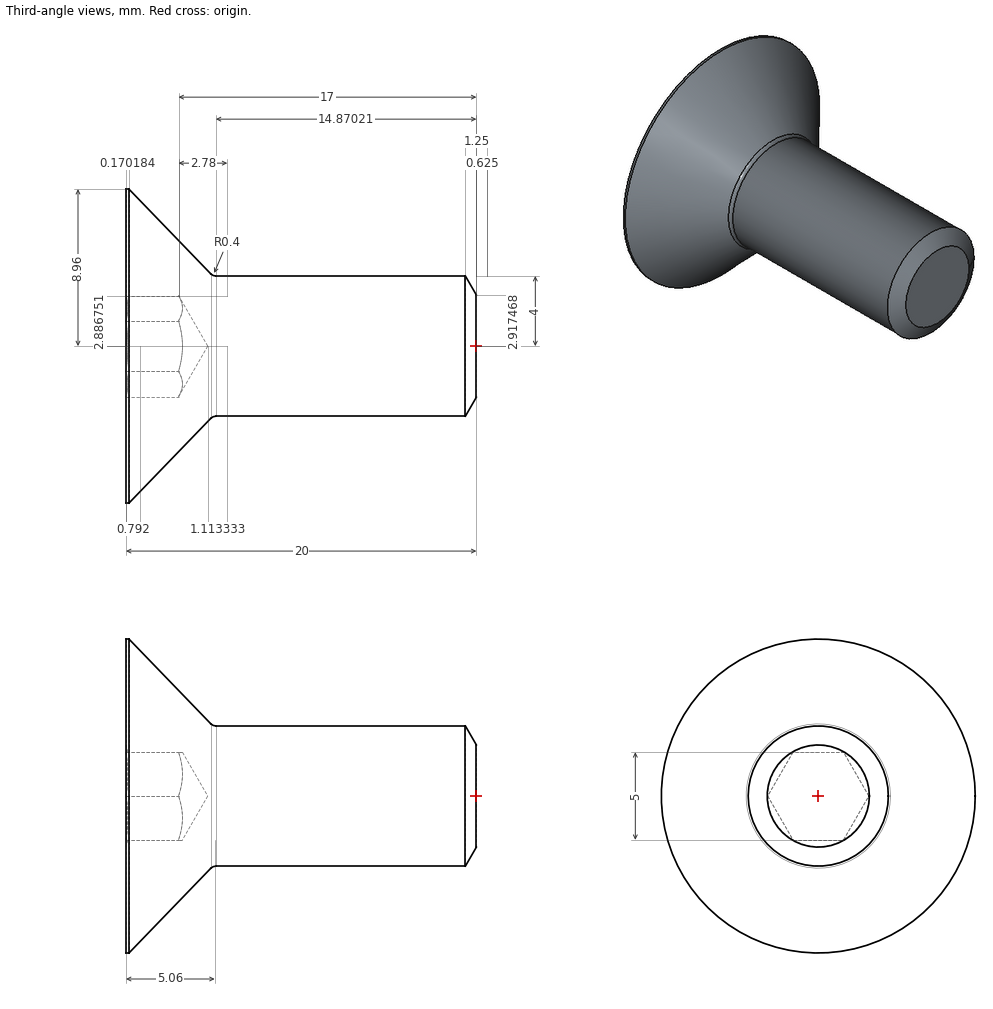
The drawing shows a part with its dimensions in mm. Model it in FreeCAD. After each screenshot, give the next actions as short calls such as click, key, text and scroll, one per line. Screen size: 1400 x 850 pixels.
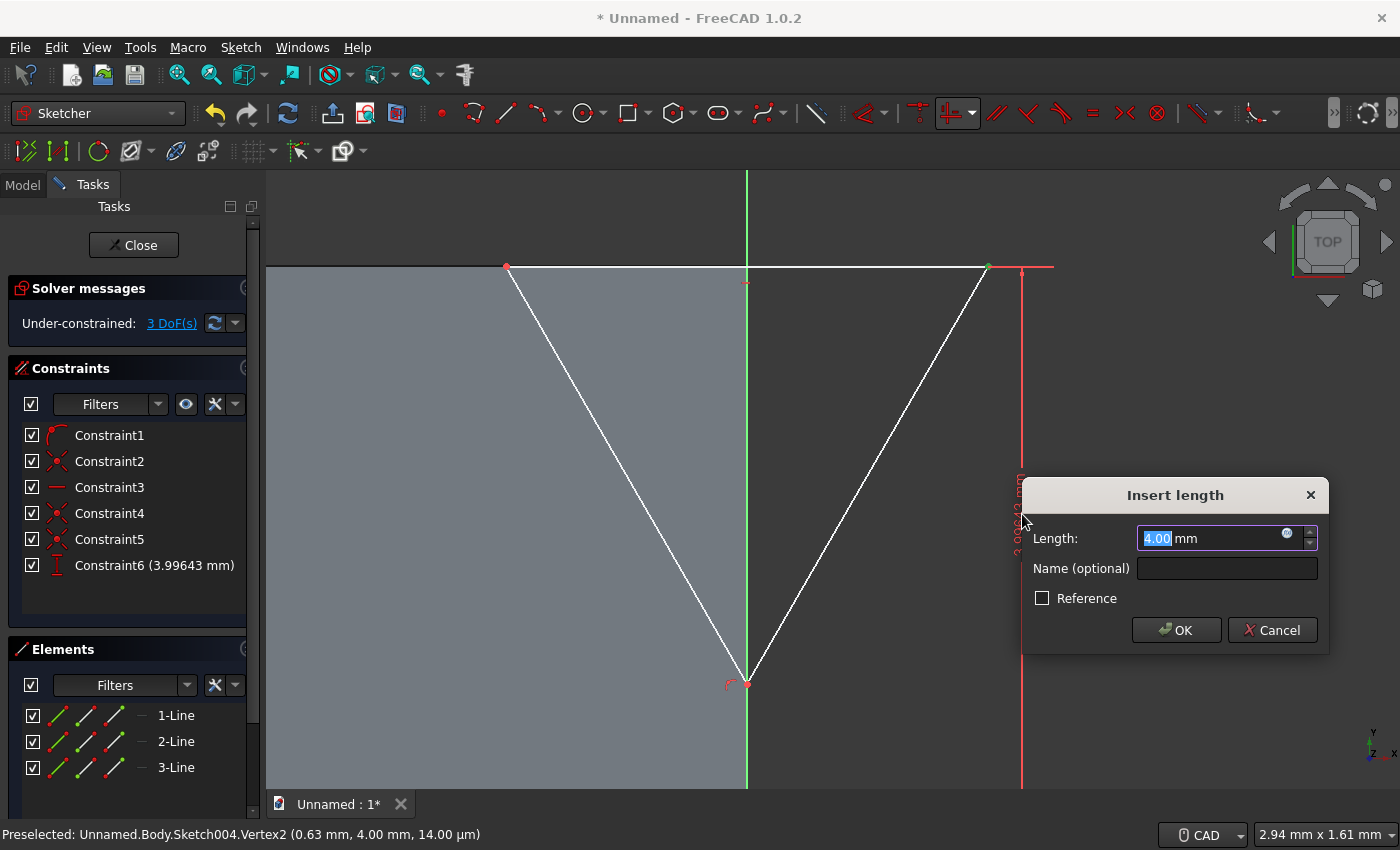
text(4)
key(Return)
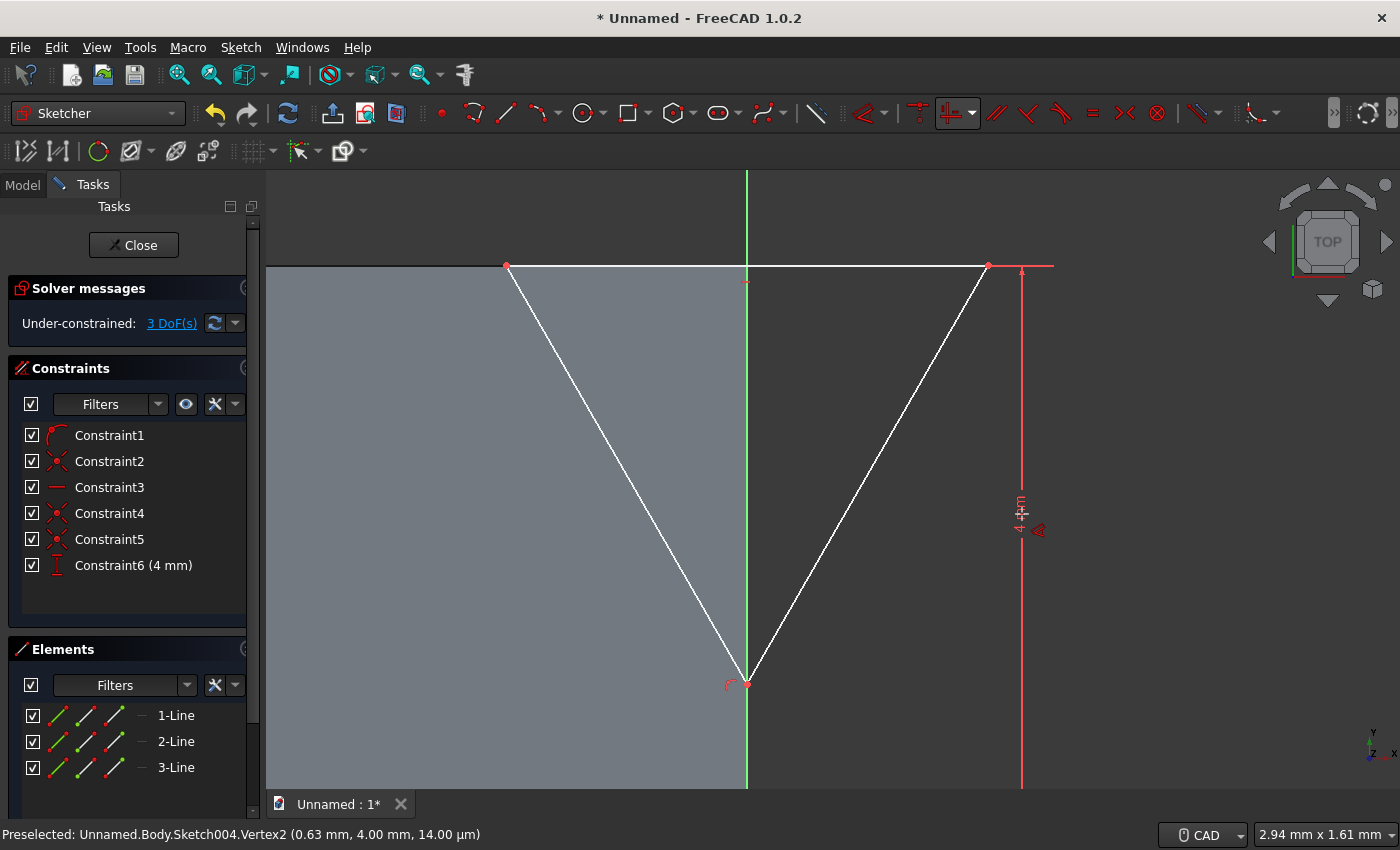
click(843, 266)
click(636, 232)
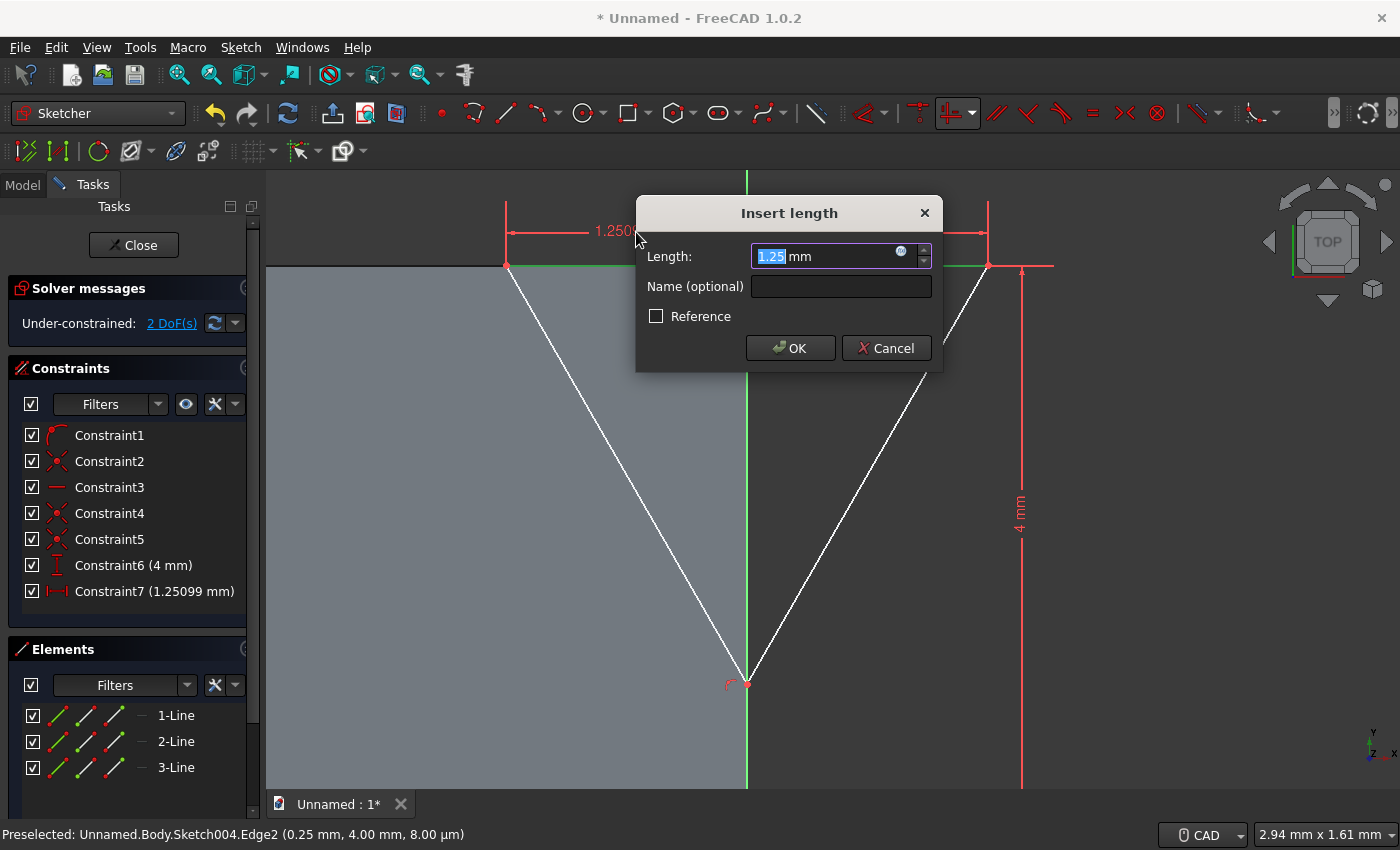
text(1.25)
key(Return)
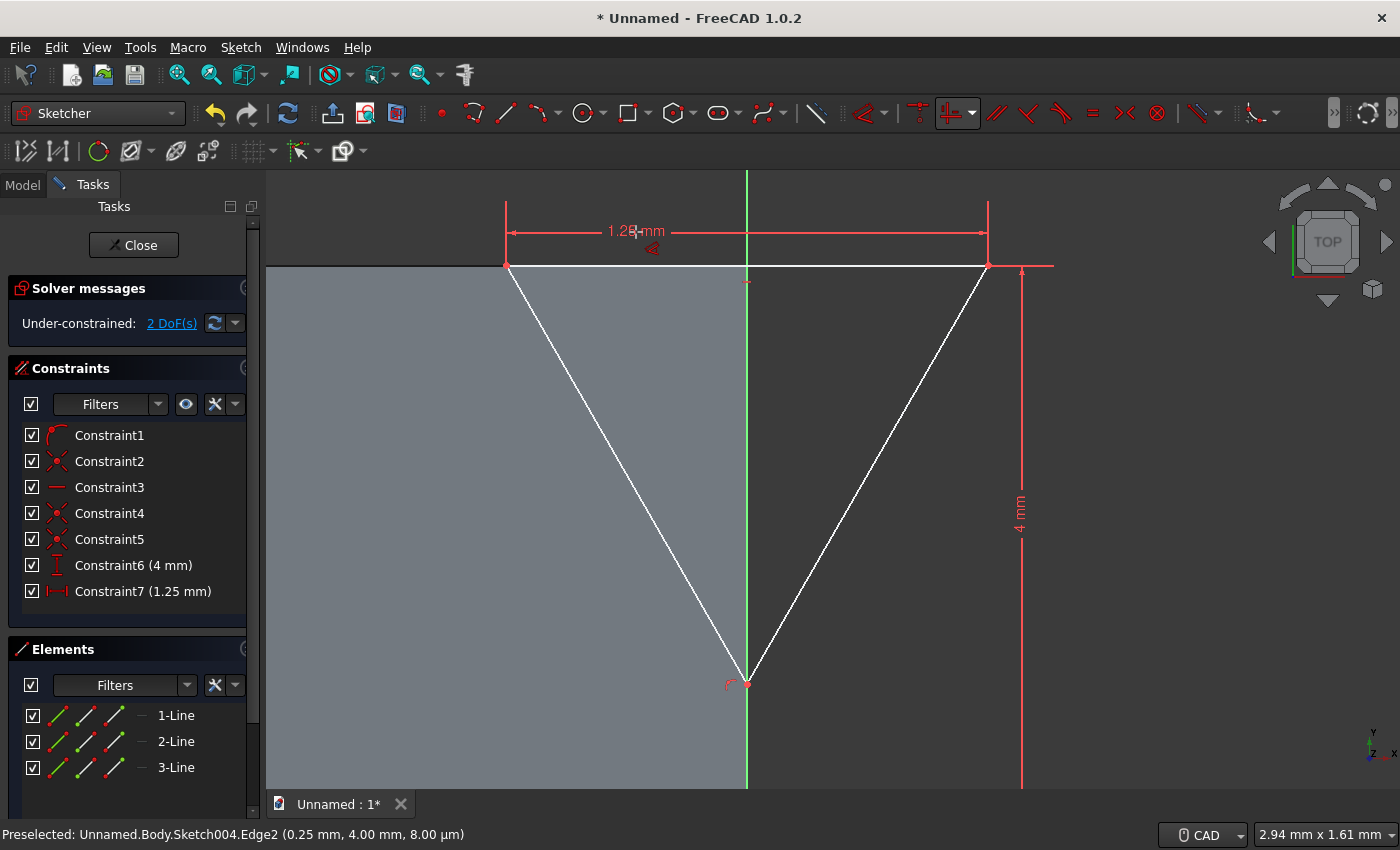
click(988, 266)
click(868, 232)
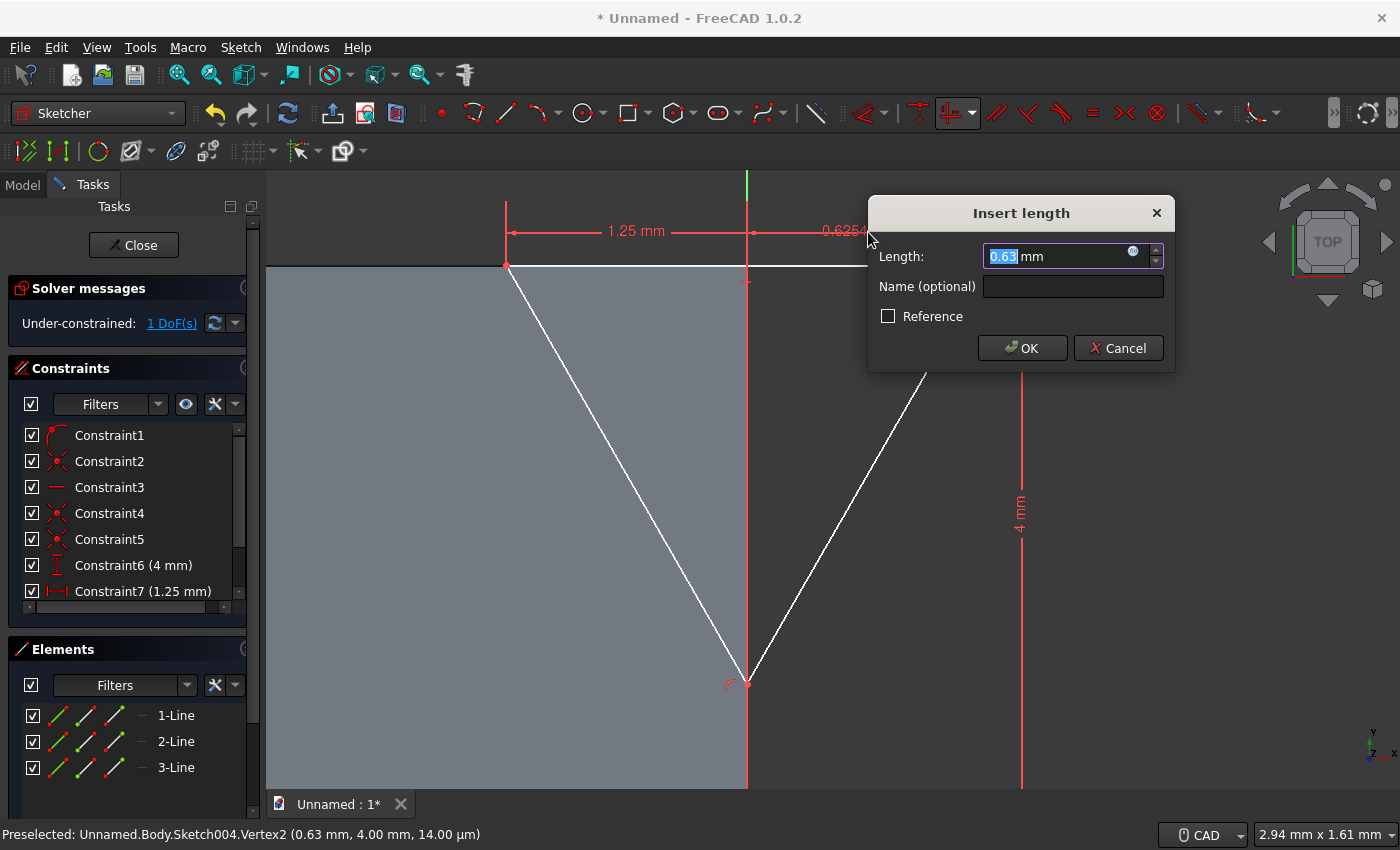
text(0.625)
key(Return)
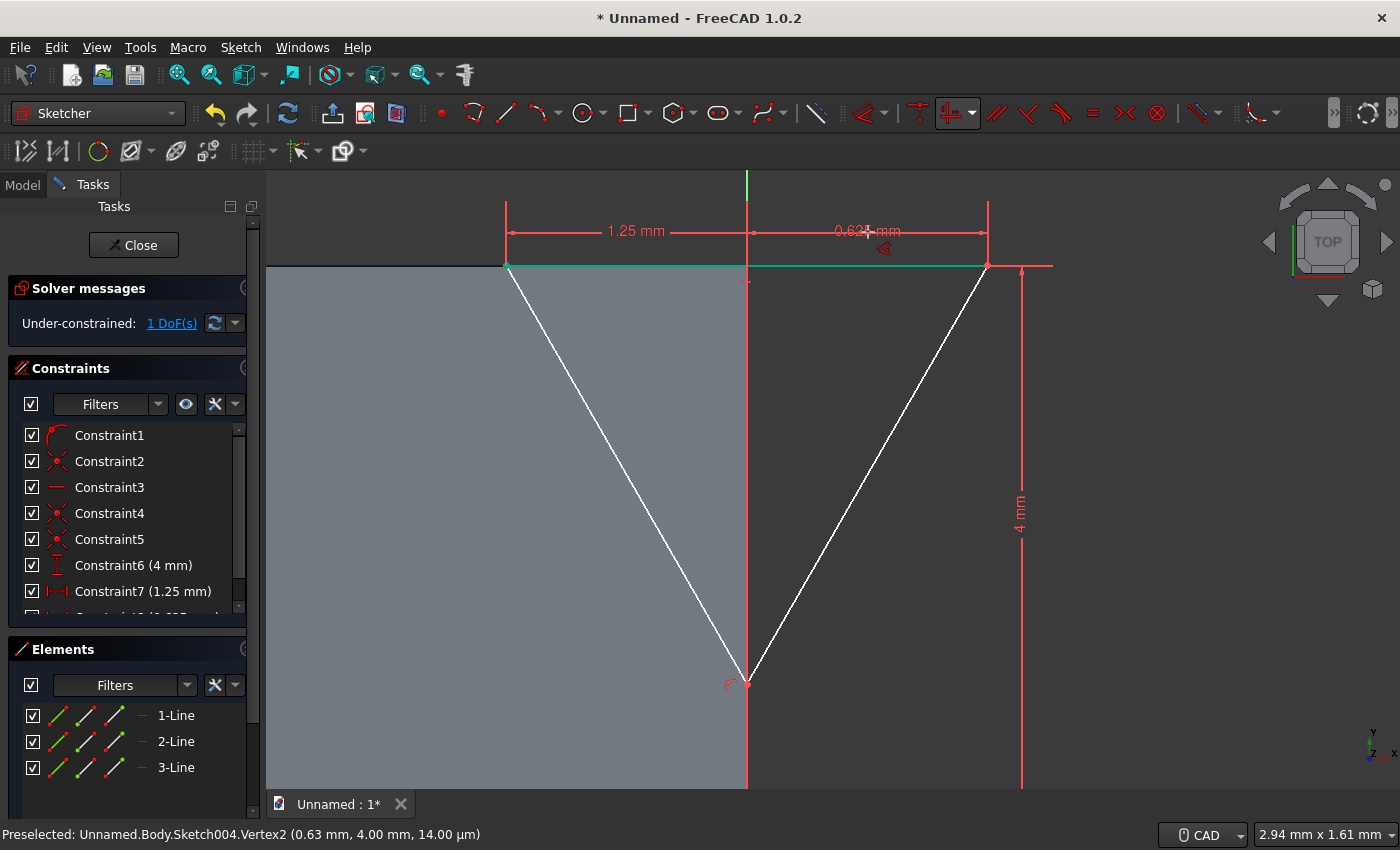
click(747, 684)
click(781, 723)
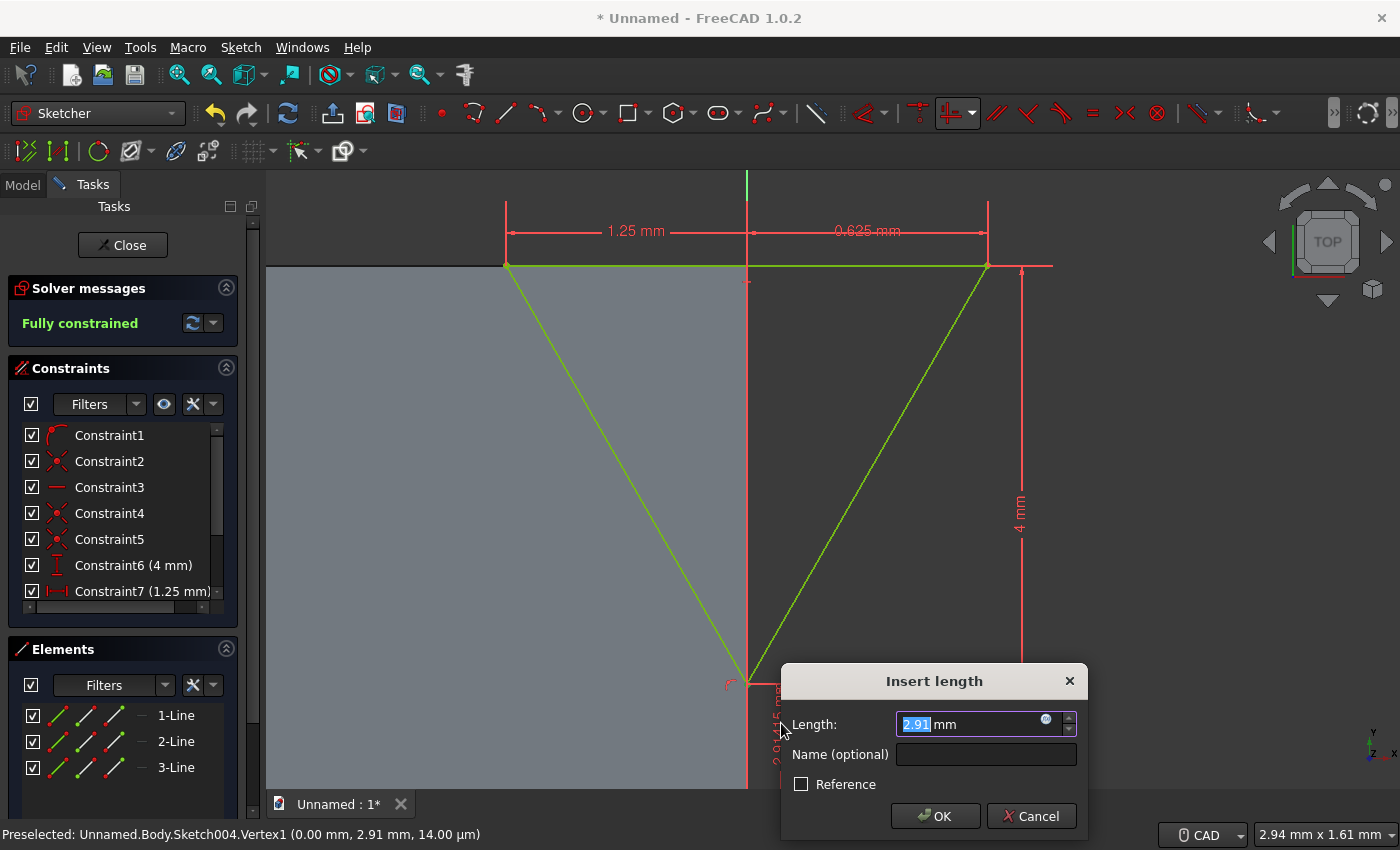
text(2.917468)
key(Return)
key(Escape)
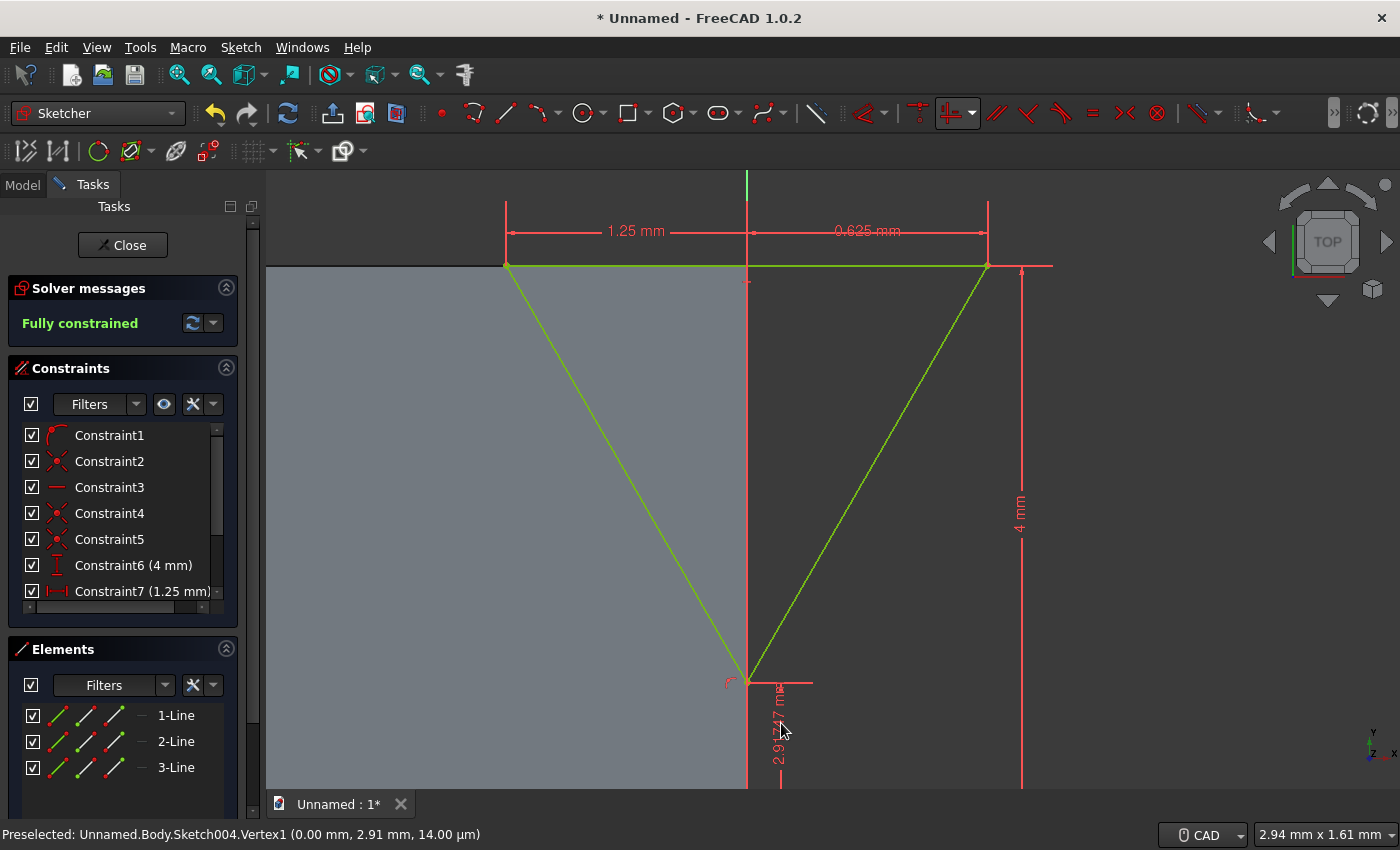
click(123, 245)